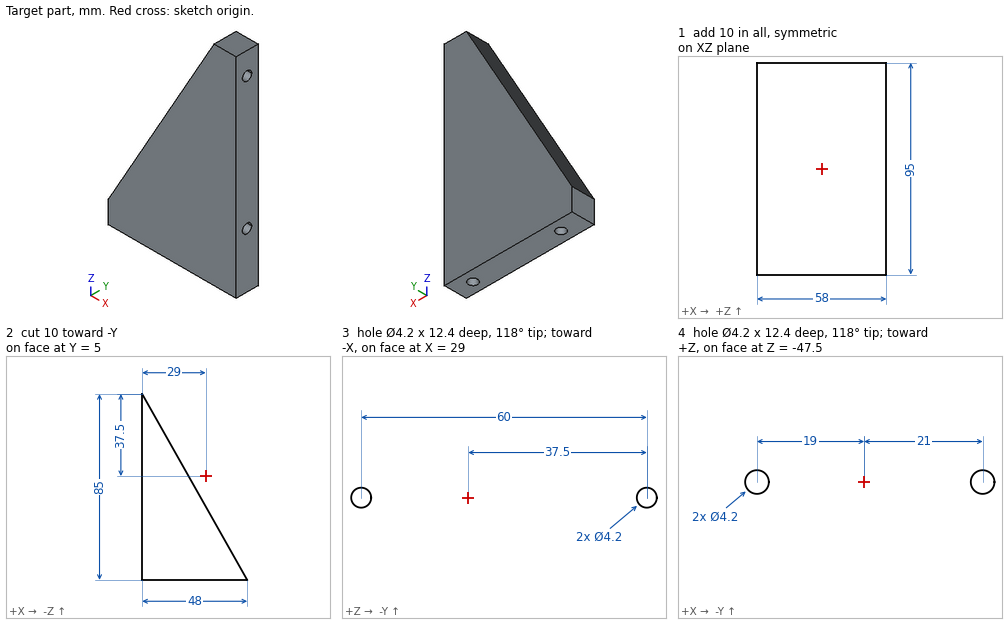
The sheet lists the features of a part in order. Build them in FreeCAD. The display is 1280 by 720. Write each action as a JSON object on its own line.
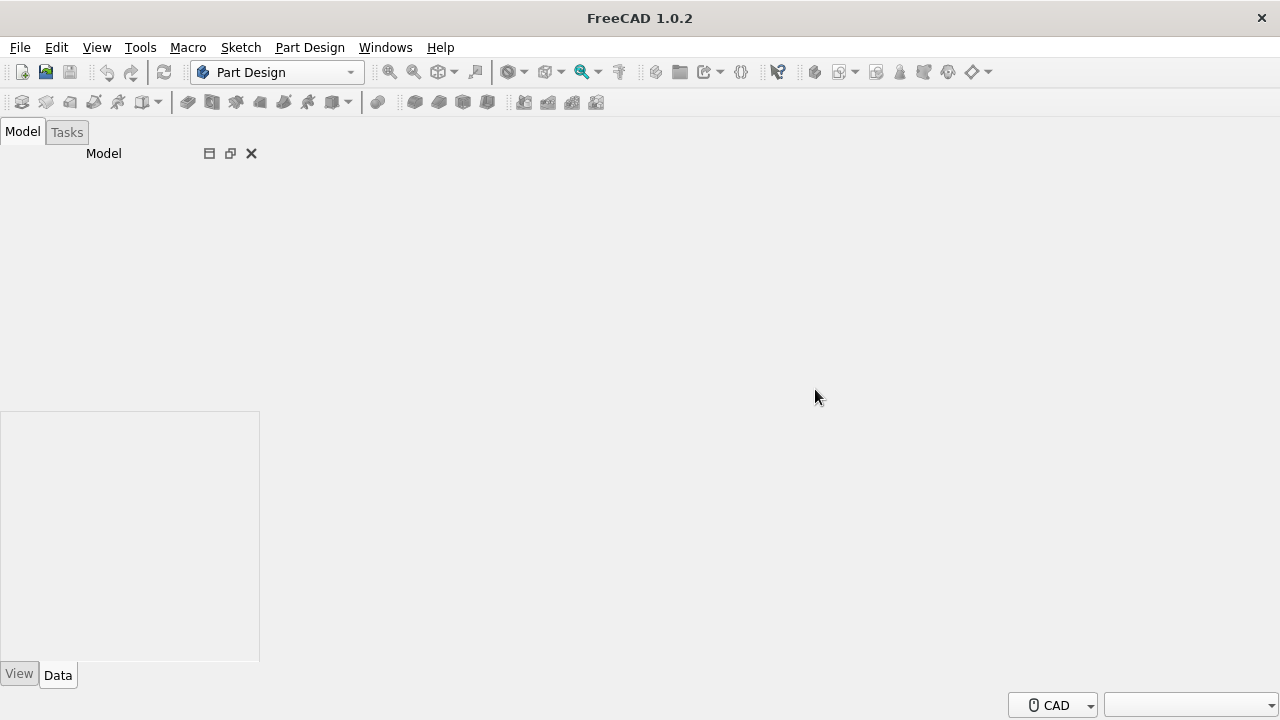
{"action": "left_click", "coordinate": [22, 72]}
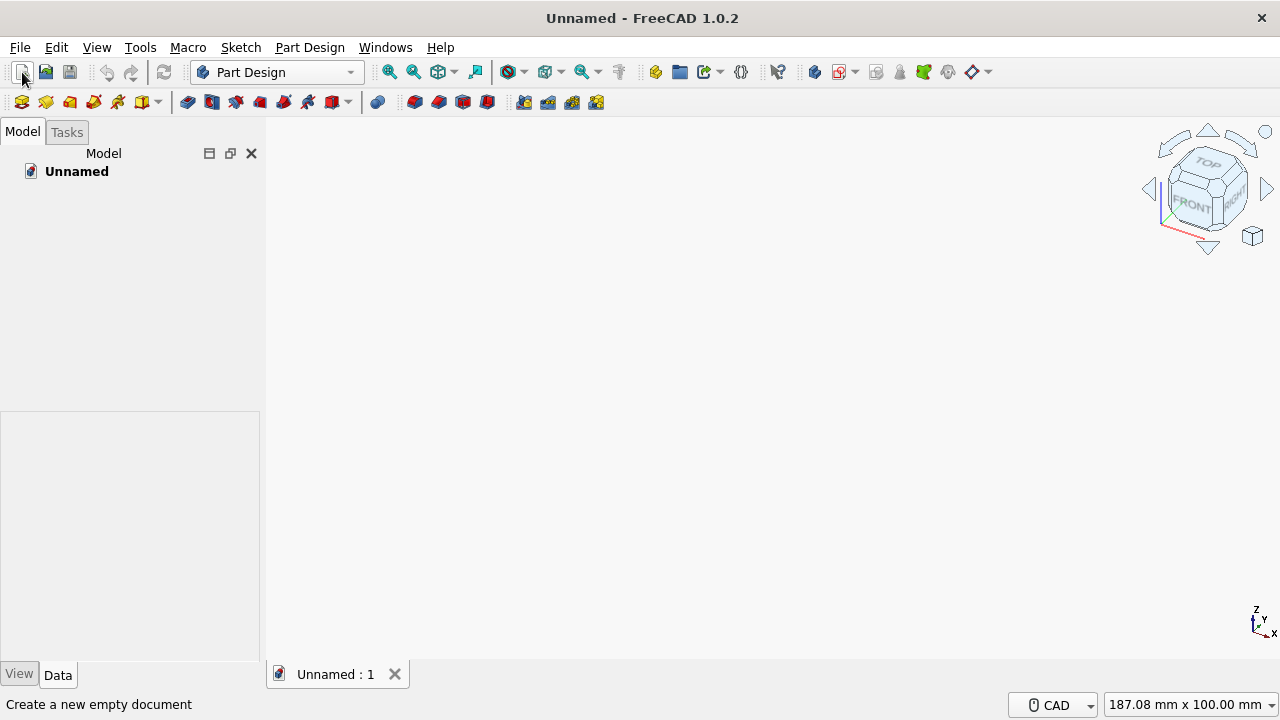
{"action": "left_click", "coordinate": [840, 72]}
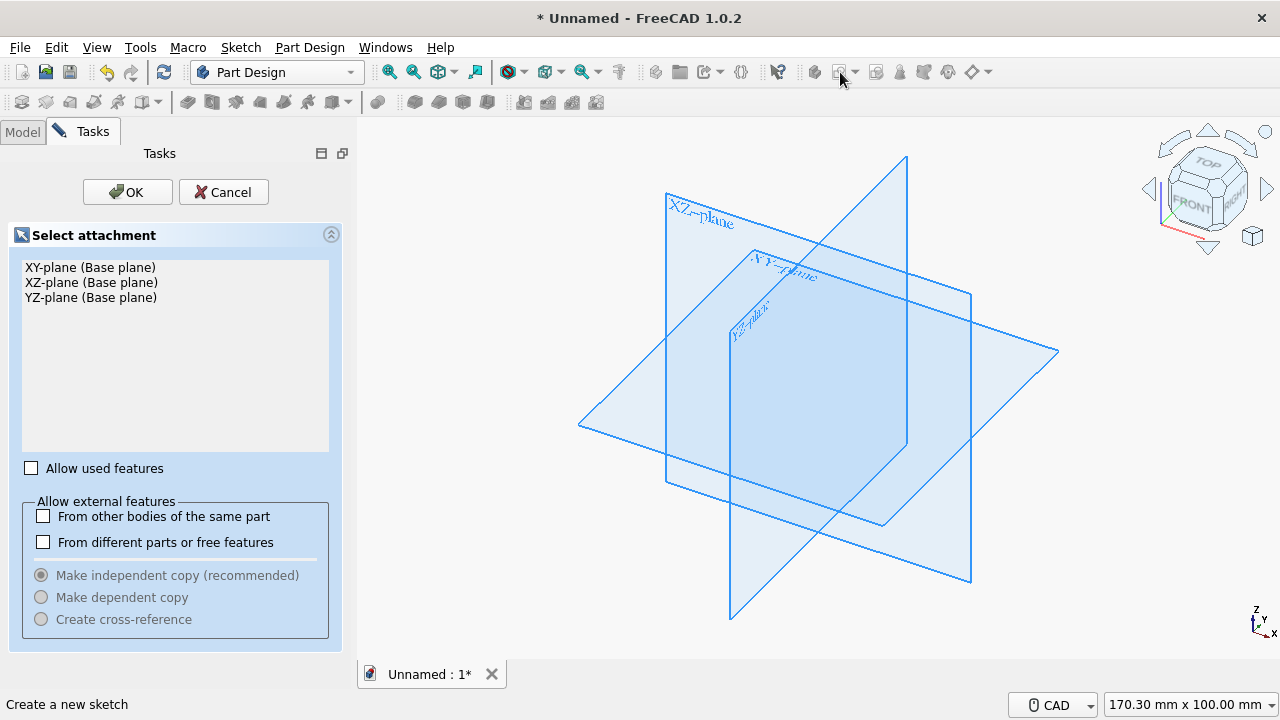
{"action": "left_click", "coordinate": [82, 282]}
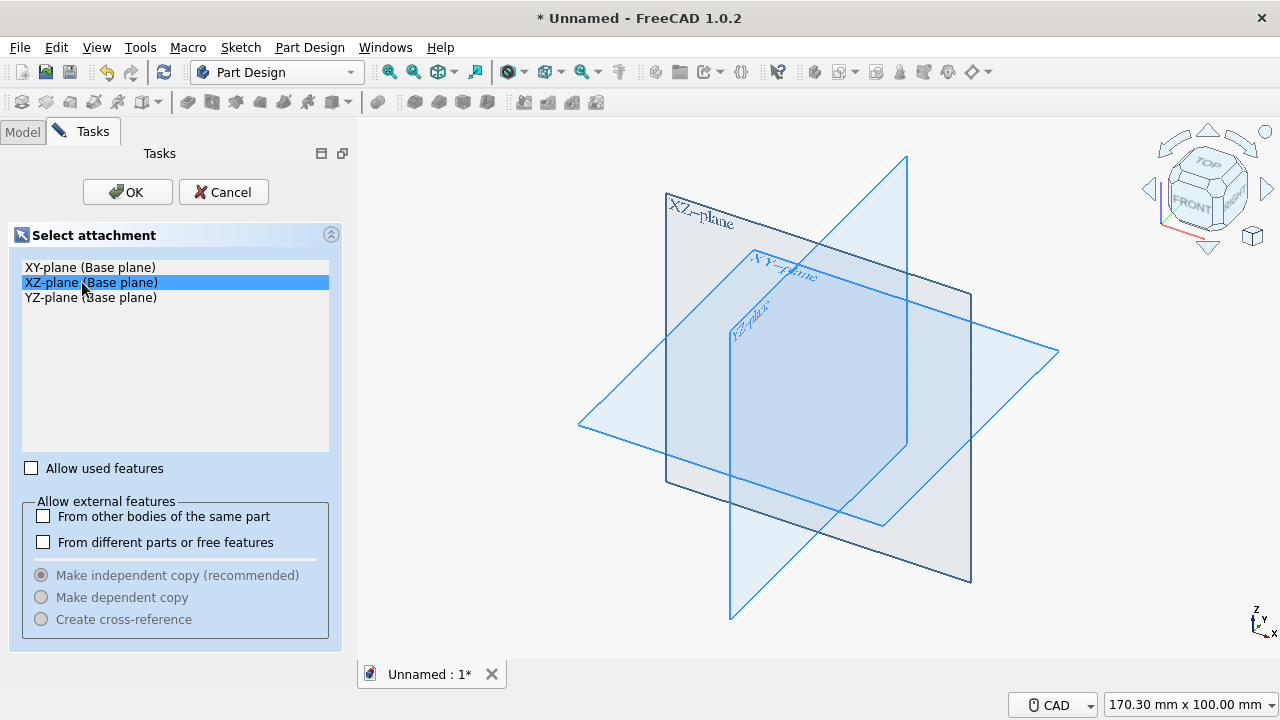
{"action": "left_click", "coordinate": [128, 192]}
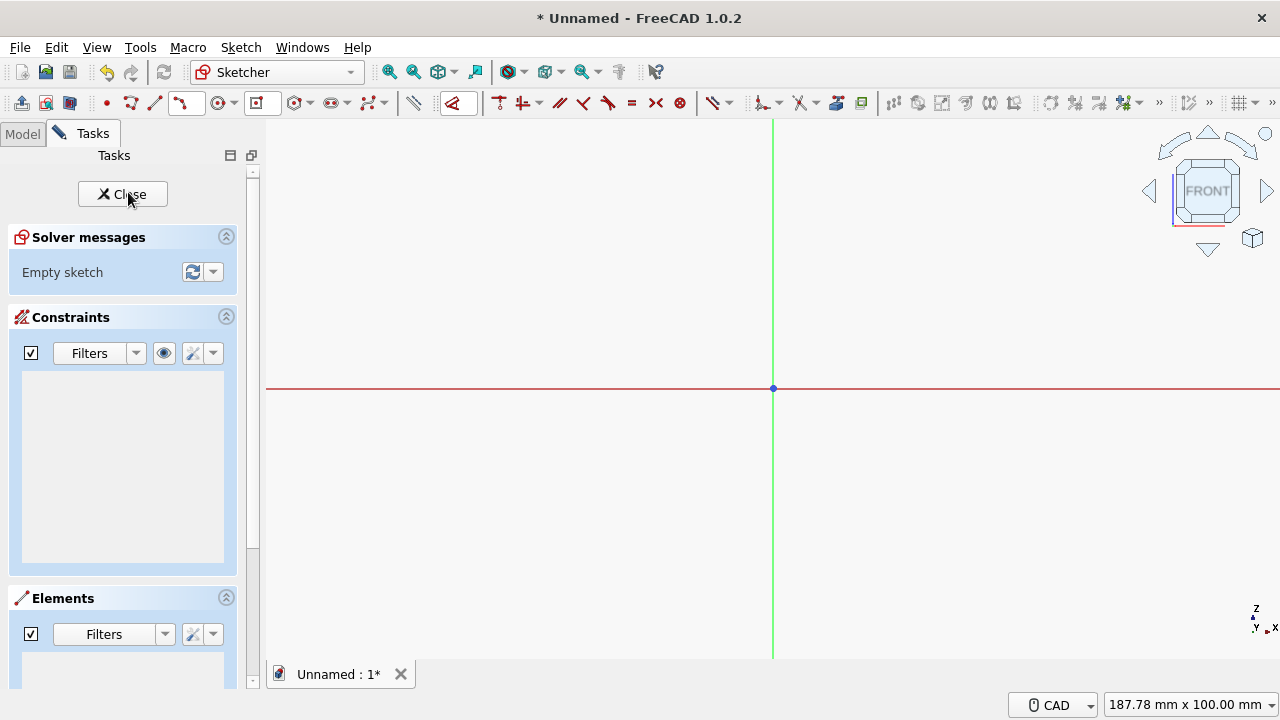
{"action": "scroll", "coordinate": [565, 389], "scroll_direction": "down", "scroll_amount": 2}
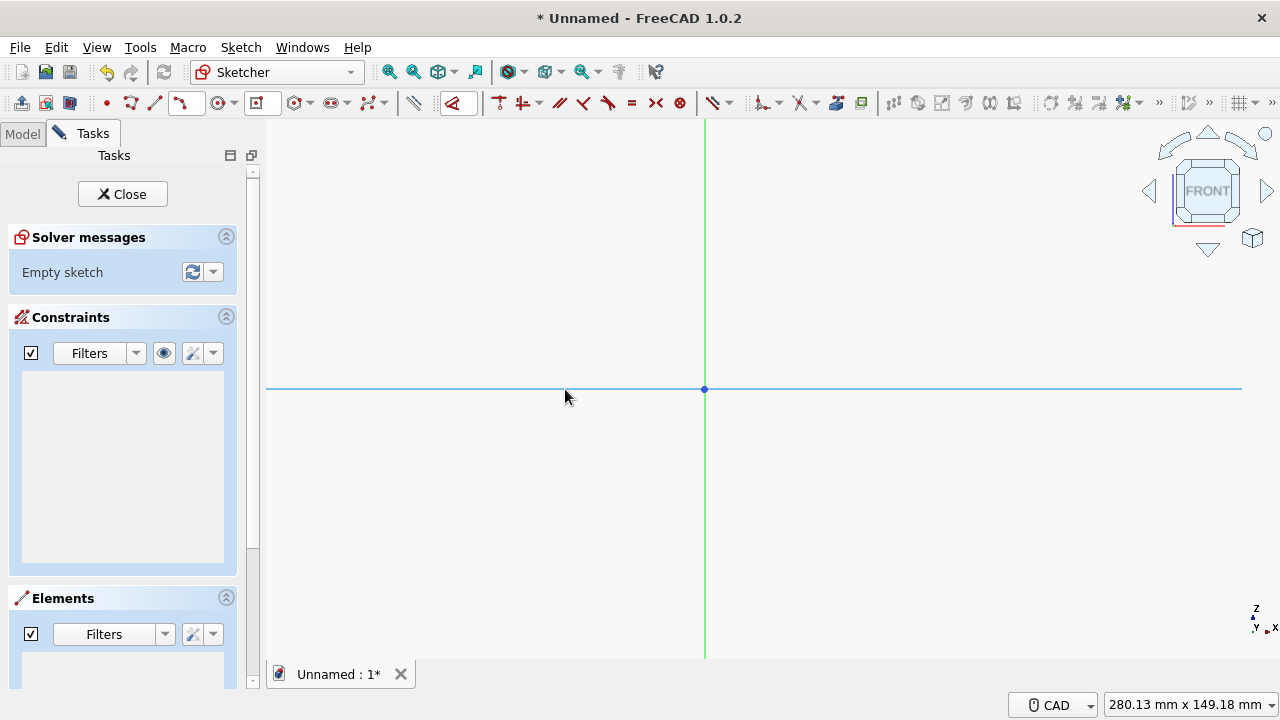
{"action": "left_click", "coordinate": [256, 104]}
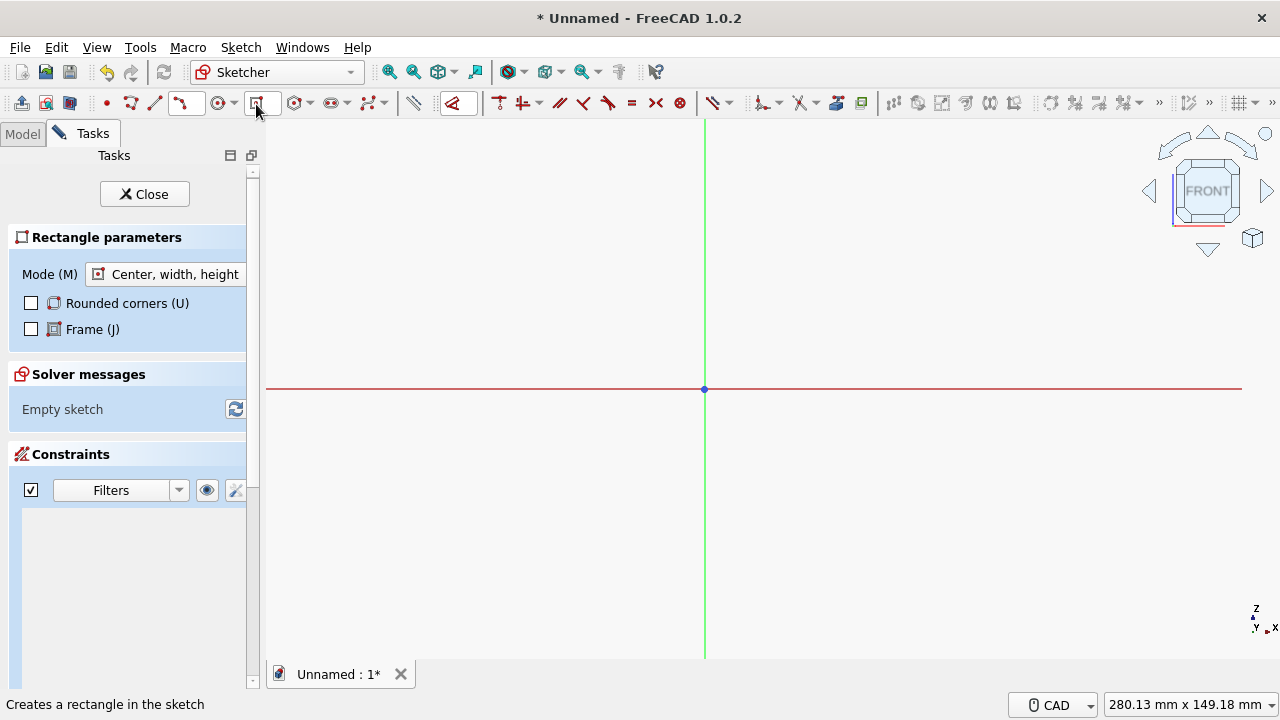
{"action": "left_click", "coordinate": [705, 389]}
{"action": "left_click", "coordinate": [809, 217]}
{"action": "key", "text": "Escape"}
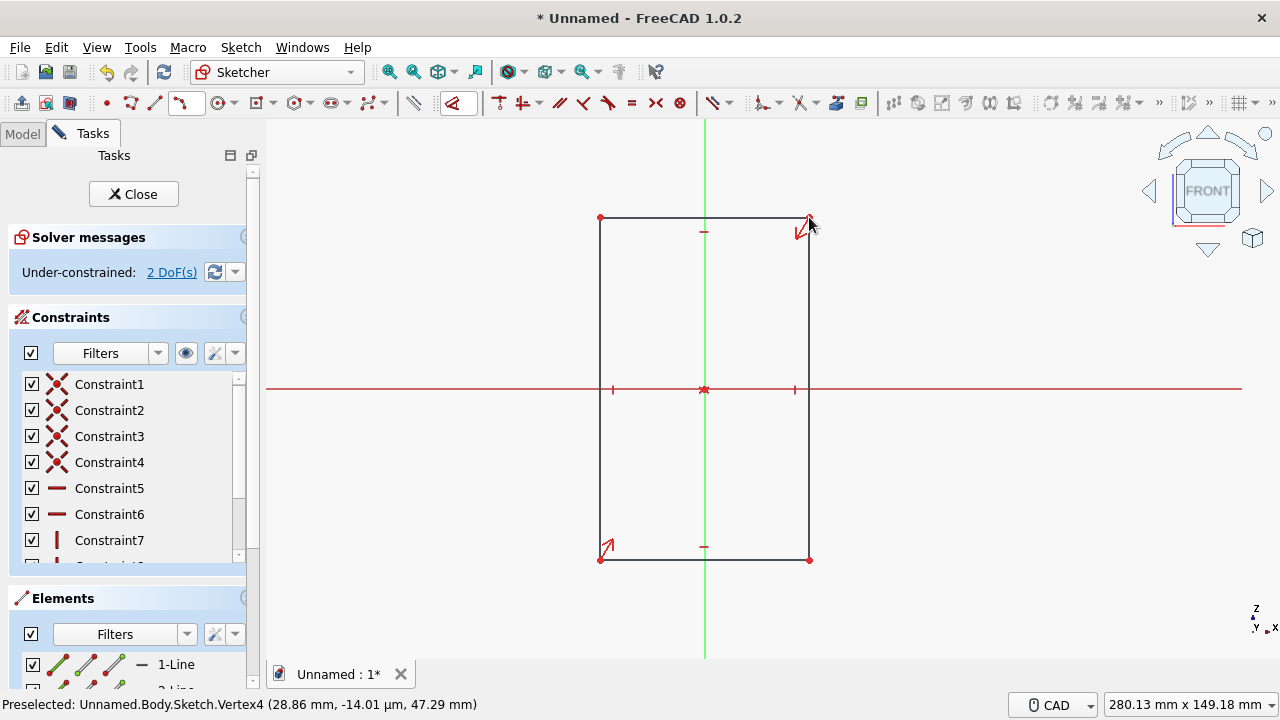
{"action": "left_click", "coordinate": [452, 104]}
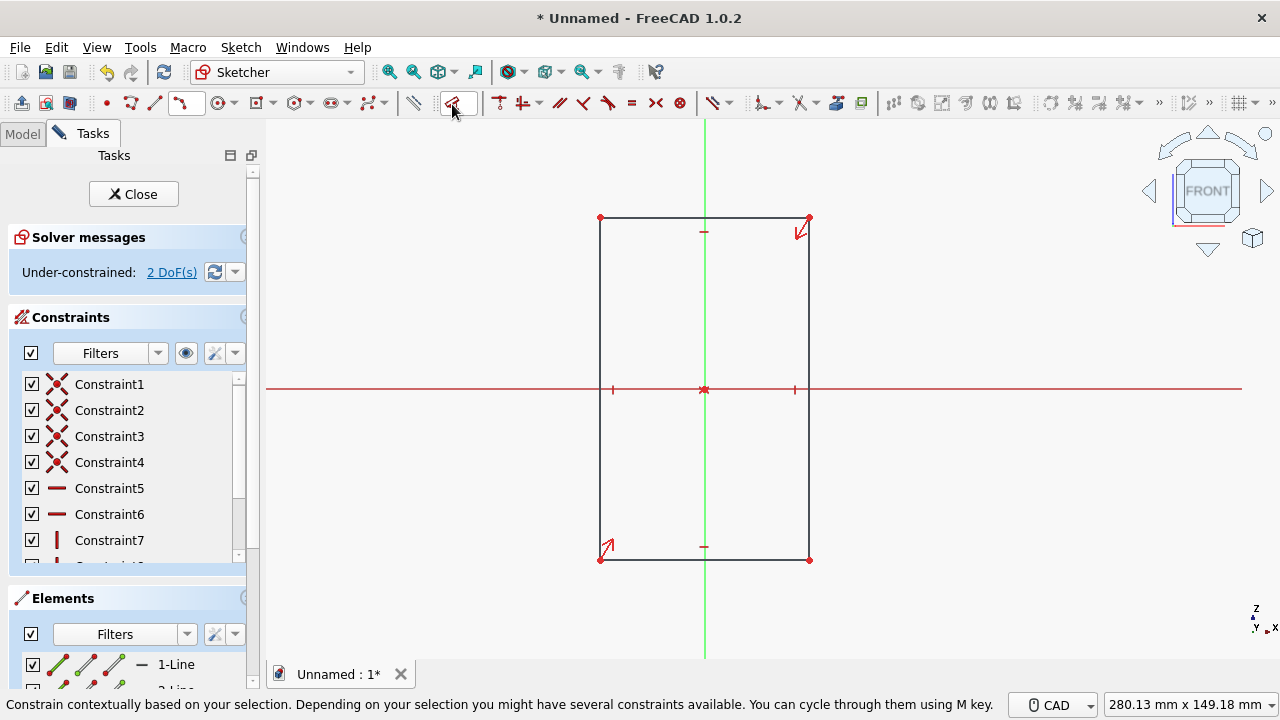
{"action": "left_click", "coordinate": [663, 560]}
{"action": "left_click", "coordinate": [656, 594]}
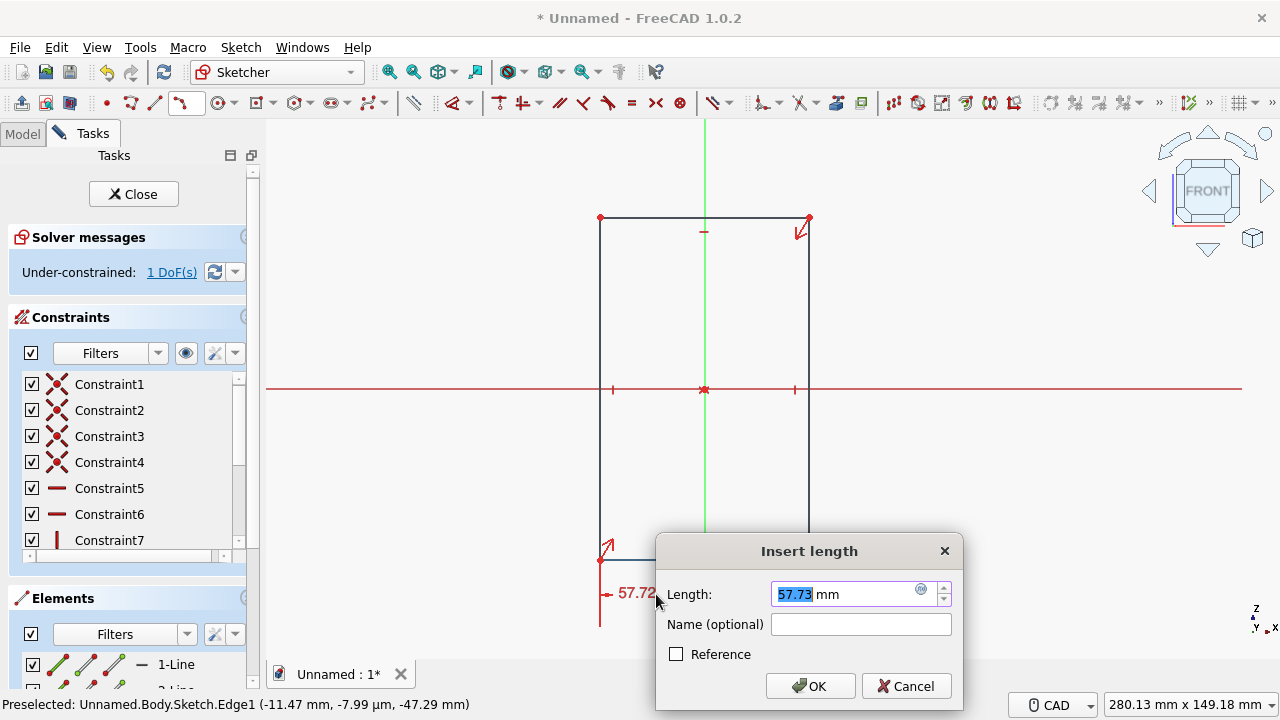
{"action": "type", "text": "58"}
{"action": "key", "text": "Return"}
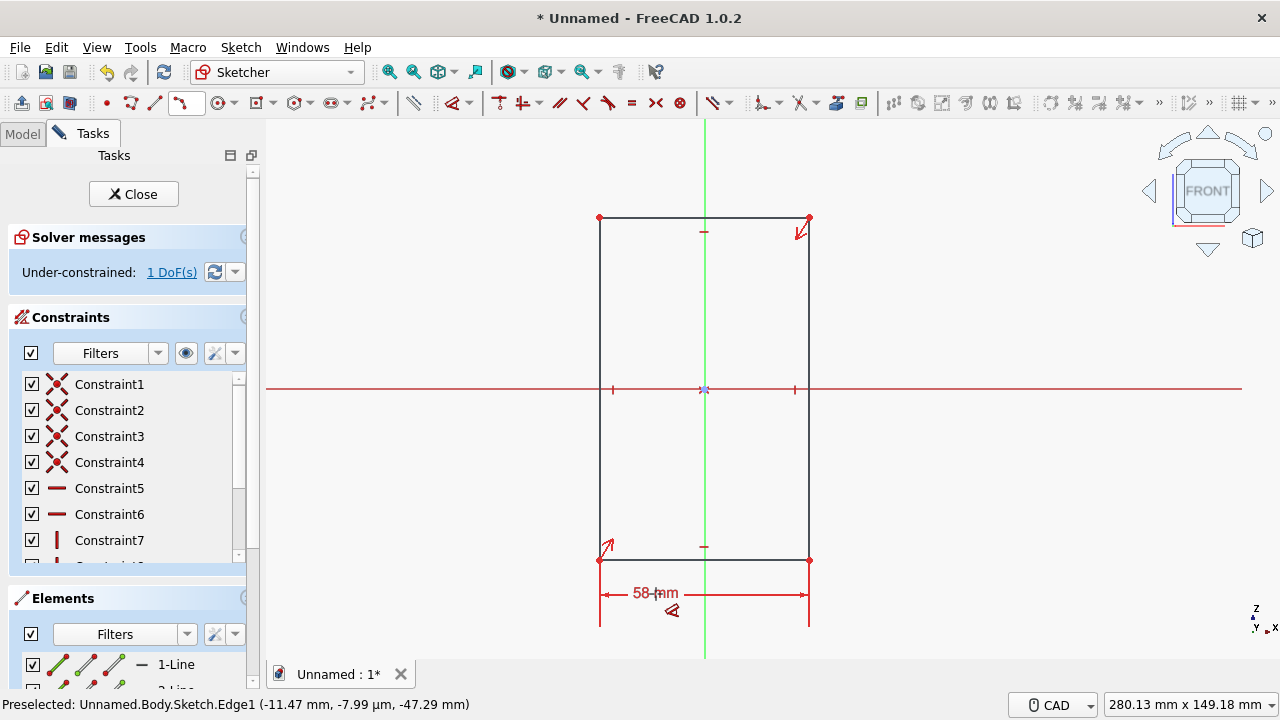
{"action": "left_click", "coordinate": [809, 458]}
{"action": "left_click", "coordinate": [843, 310]}